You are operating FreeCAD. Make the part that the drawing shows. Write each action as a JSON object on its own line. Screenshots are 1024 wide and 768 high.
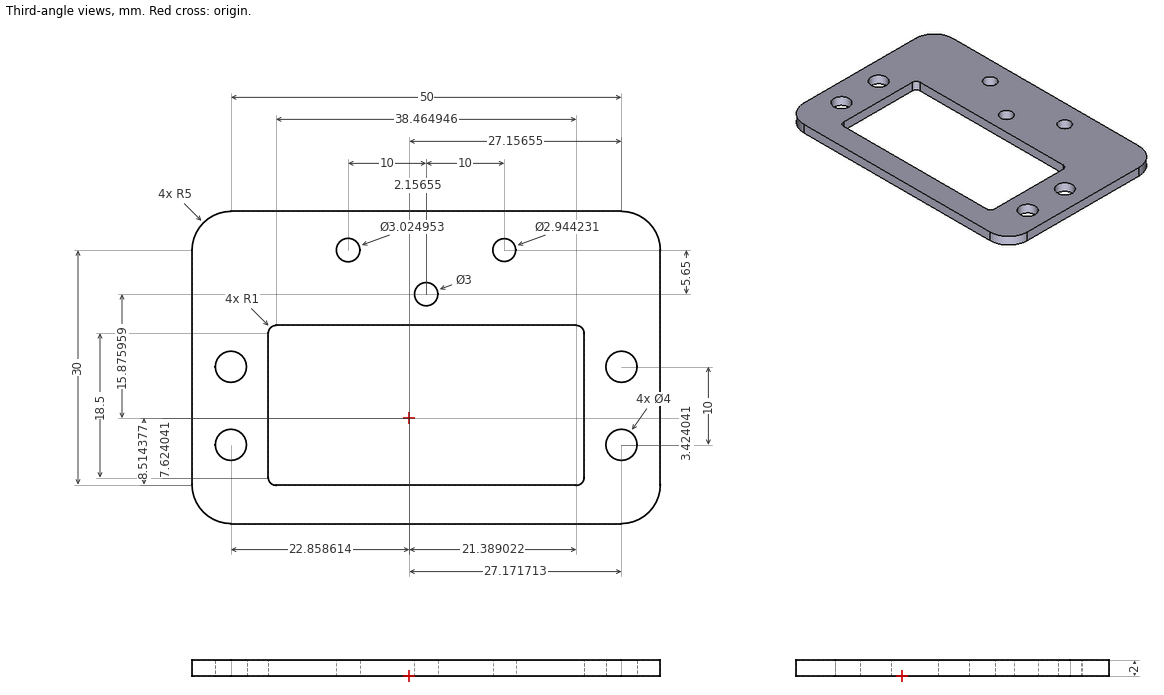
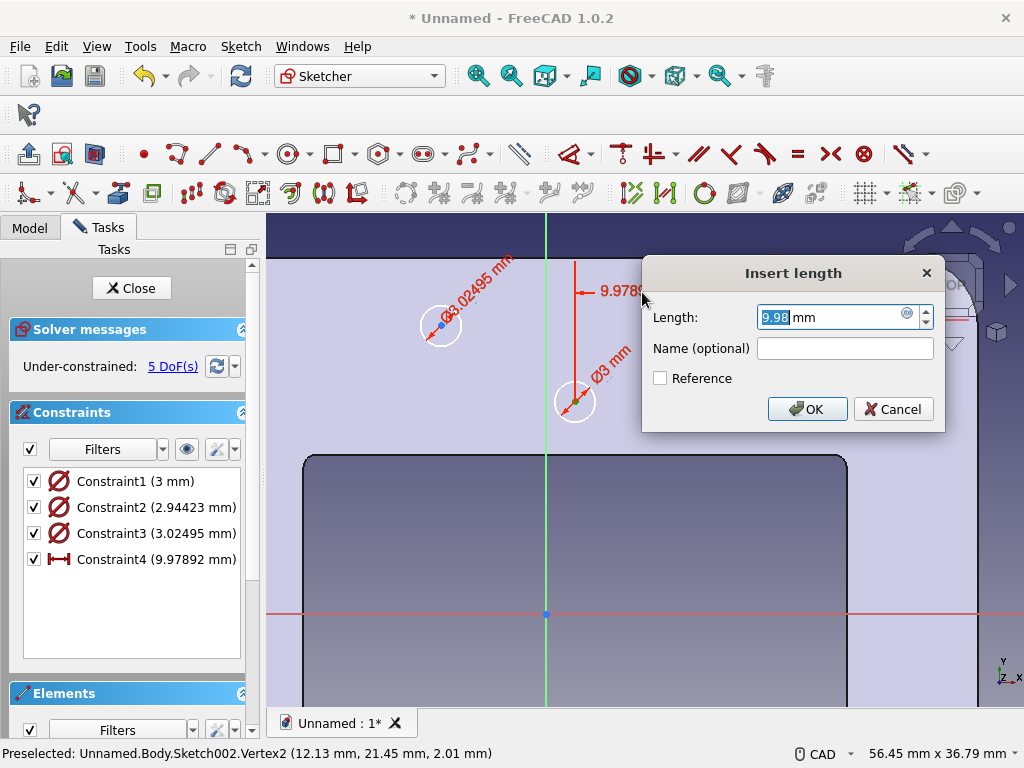
{"action": "type", "text": "10"}
{"action": "key", "text": "Return"}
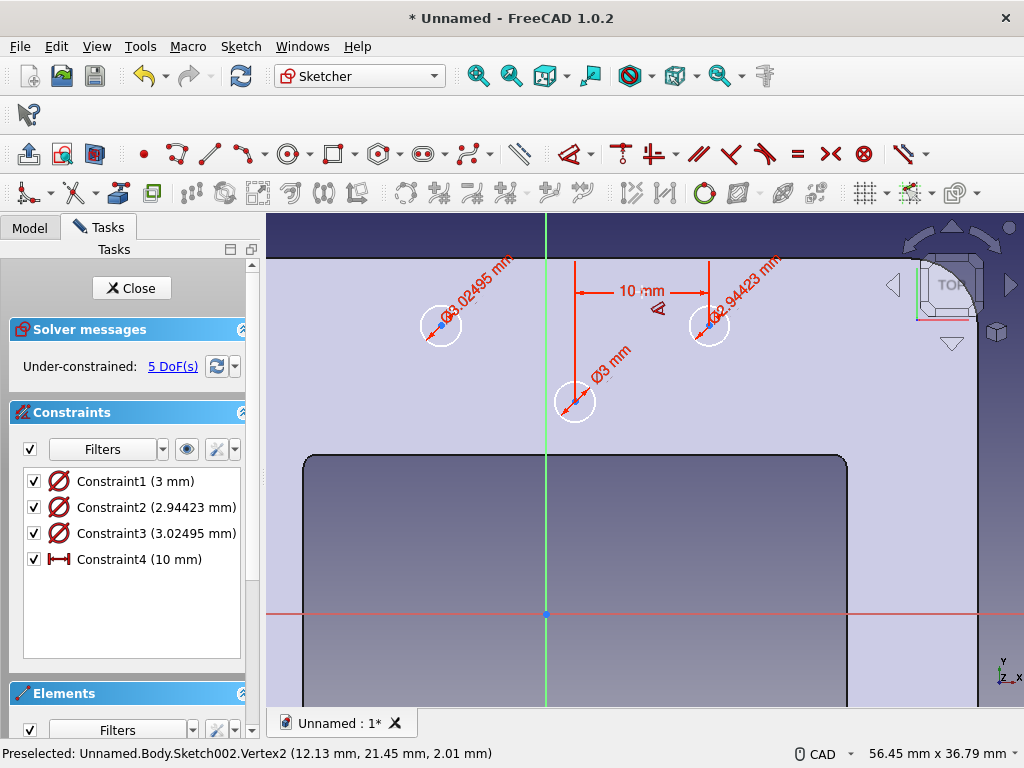
{"action": "left_click", "coordinate": [575, 402]}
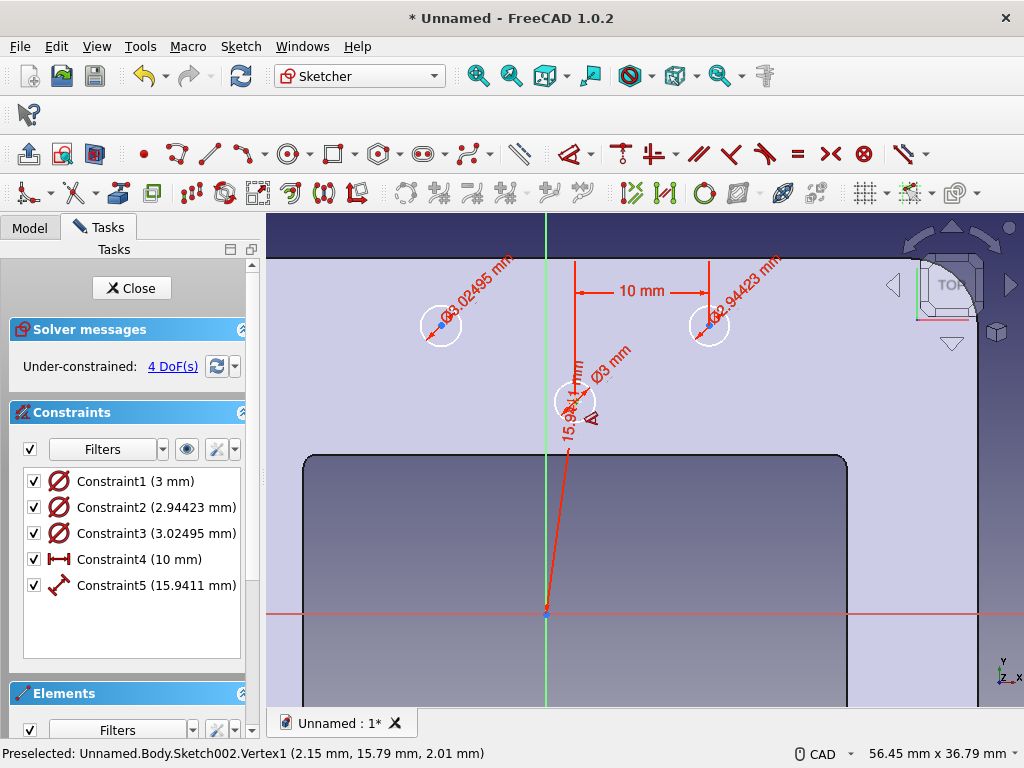
{"action": "left_click", "coordinate": [441, 326]}
{"action": "left_click", "coordinate": [508, 436]}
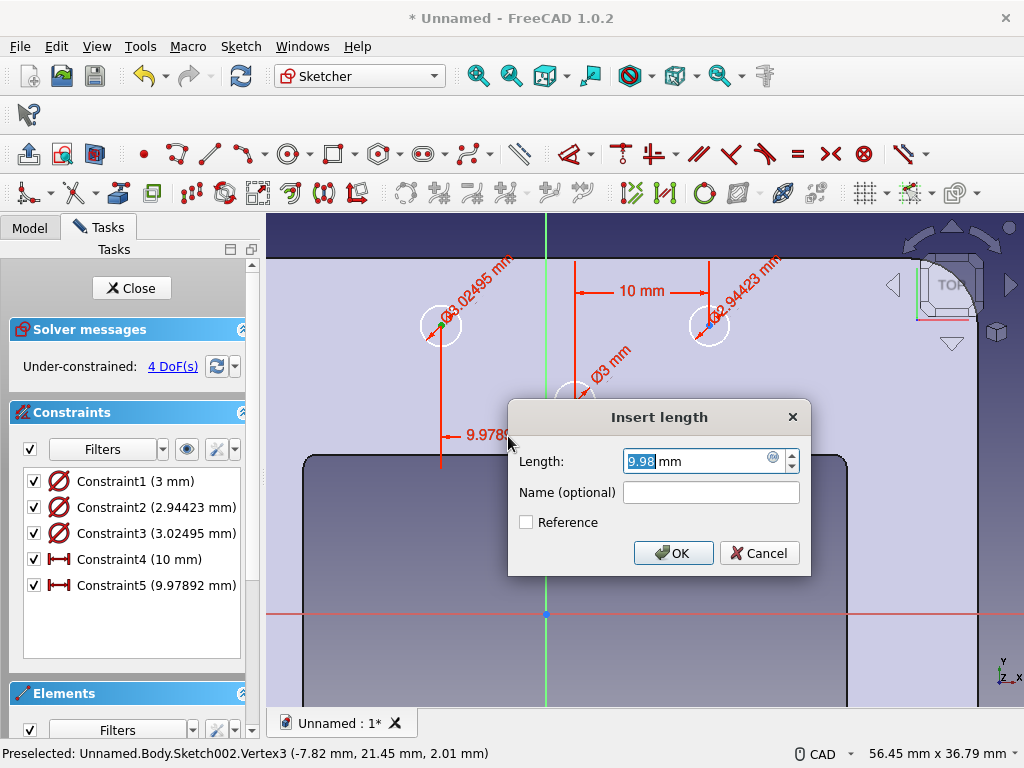
{"action": "type", "text": "10"}
{"action": "key", "text": "Return"}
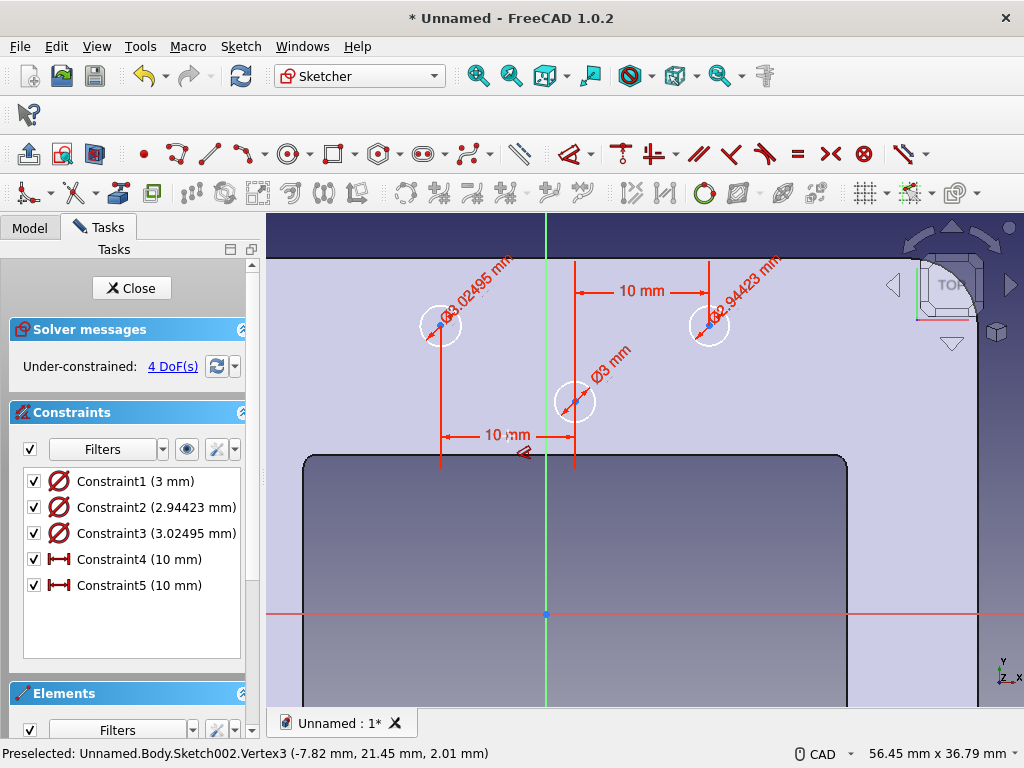
{"action": "left_click", "coordinate": [575, 402]}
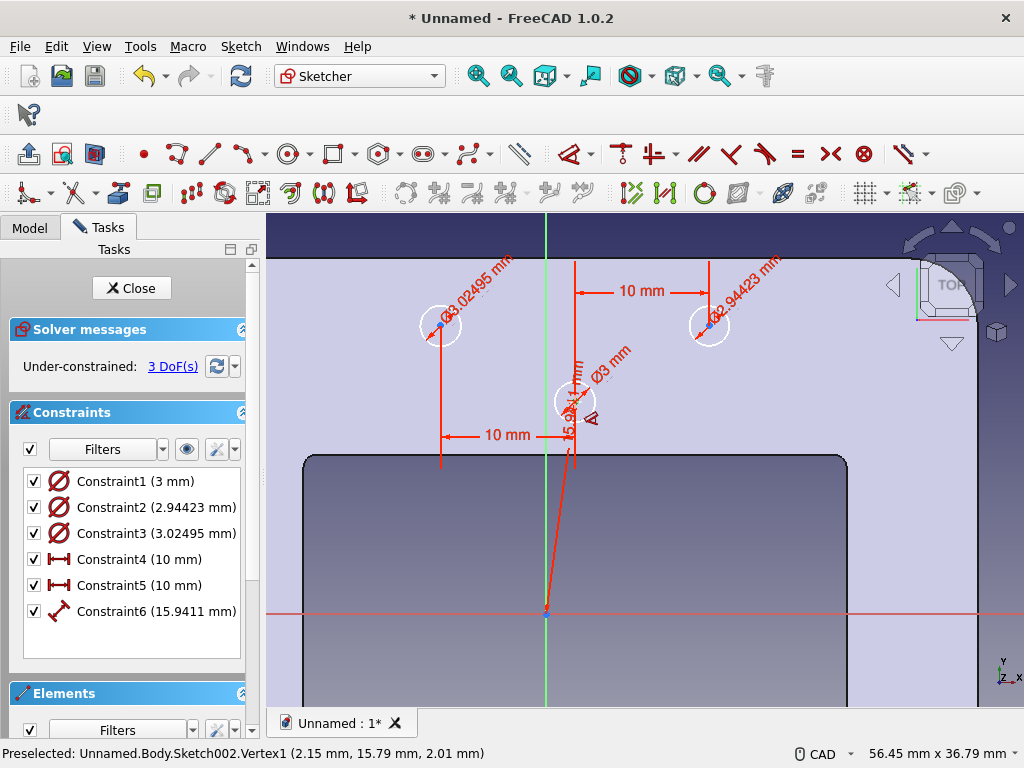
{"action": "left_click", "coordinate": [709, 326]}
{"action": "left_click", "coordinate": [743, 364]}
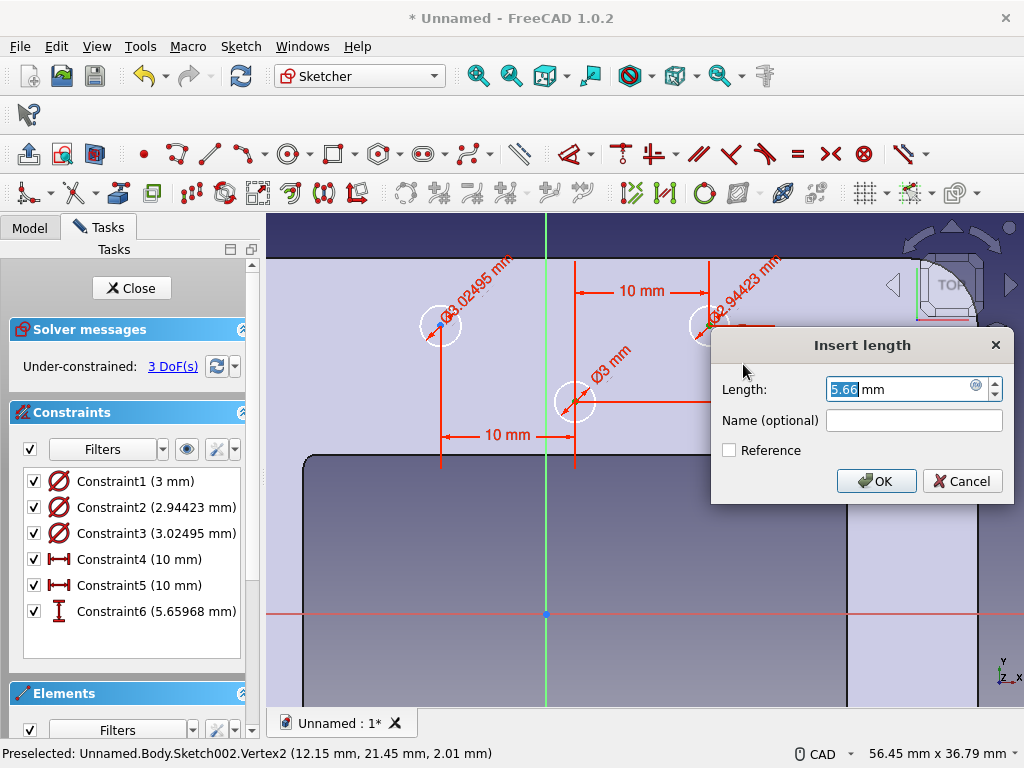
{"action": "type", "text": "5.65"}
{"action": "key", "text": "Return"}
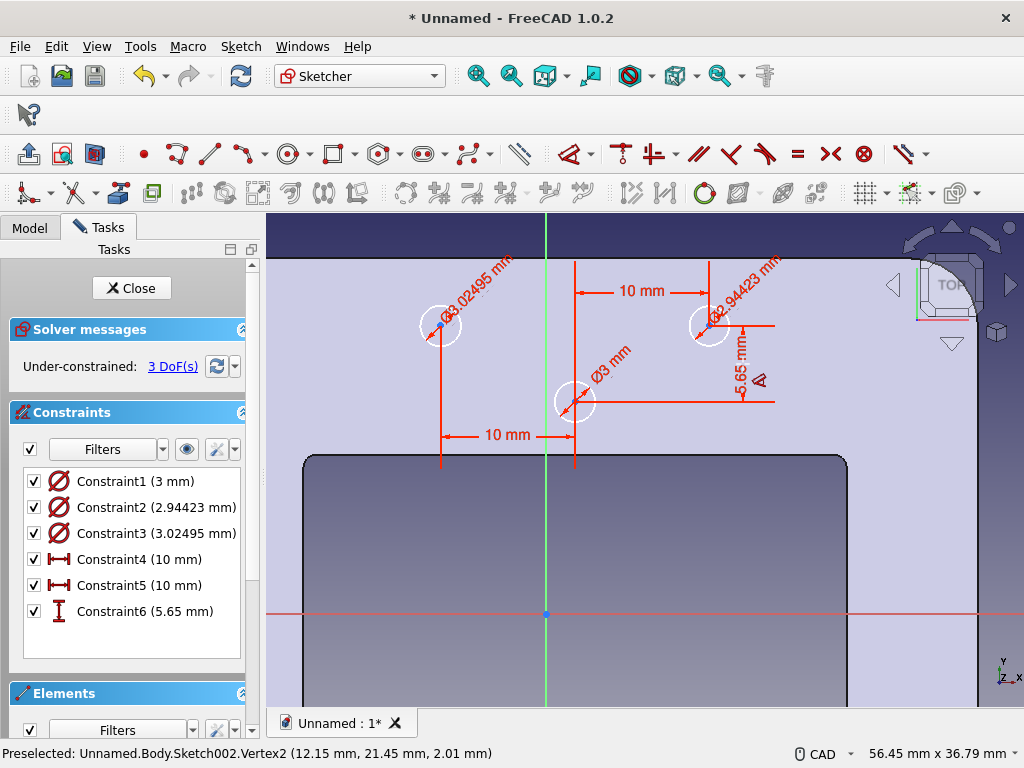
{"action": "left_click", "coordinate": [575, 402]}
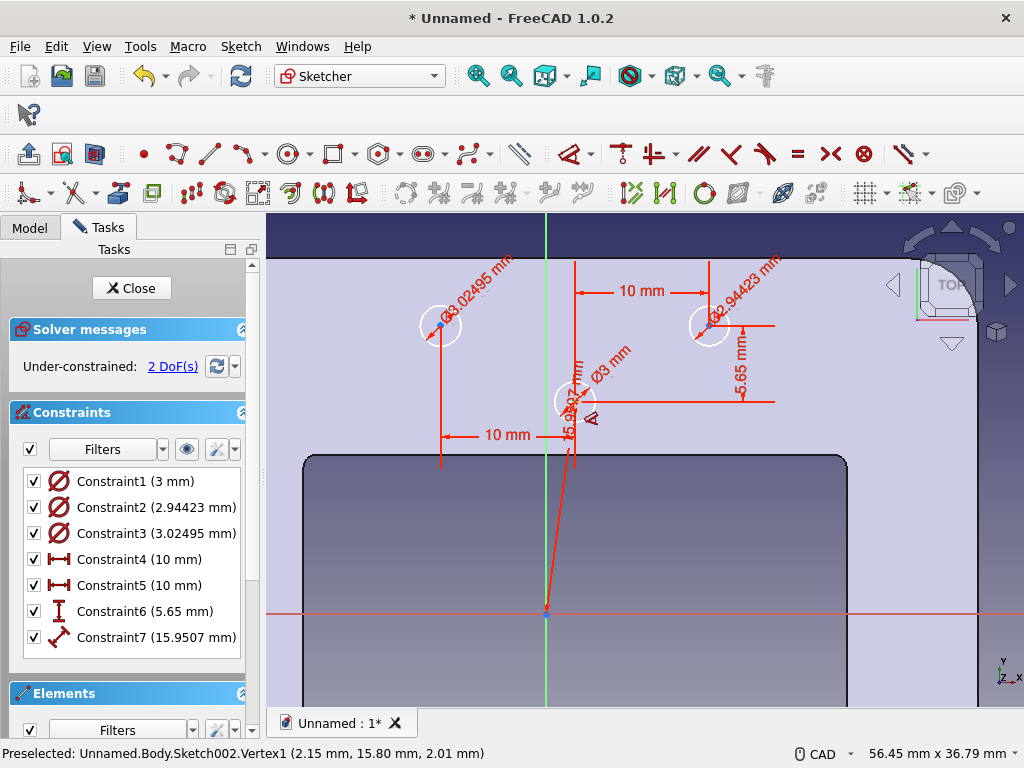
{"action": "left_click", "coordinate": [441, 326]}
{"action": "left_click", "coordinate": [407, 364]}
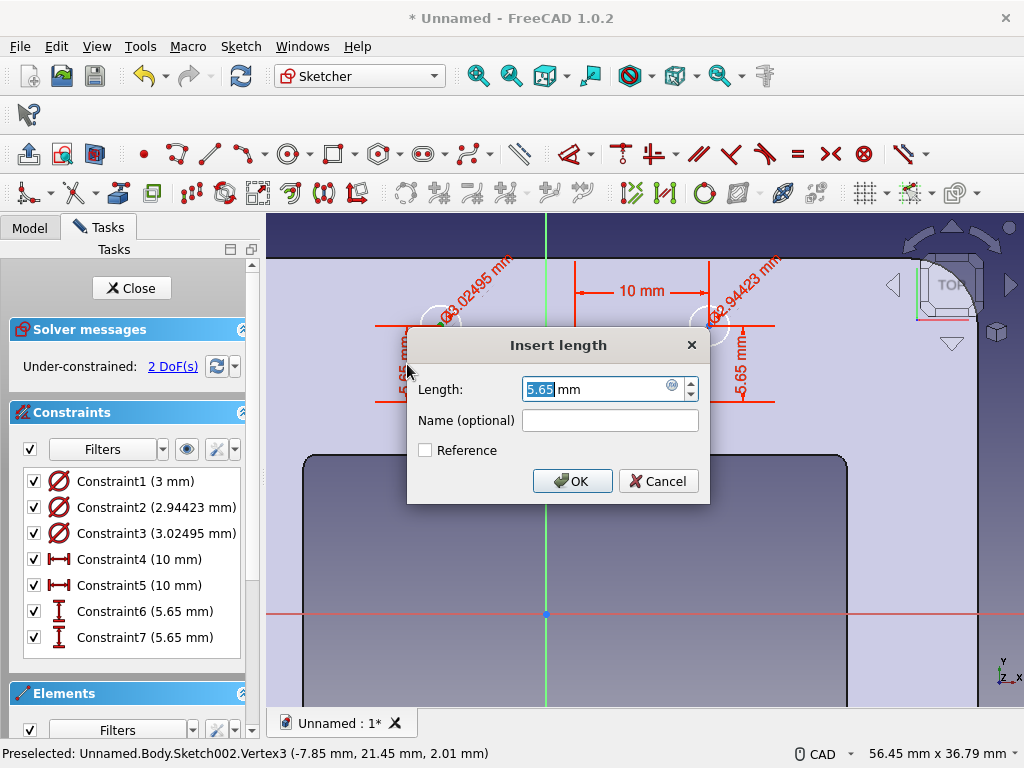
{"action": "type", "text": "5.65"}
{"action": "key", "text": "Return"}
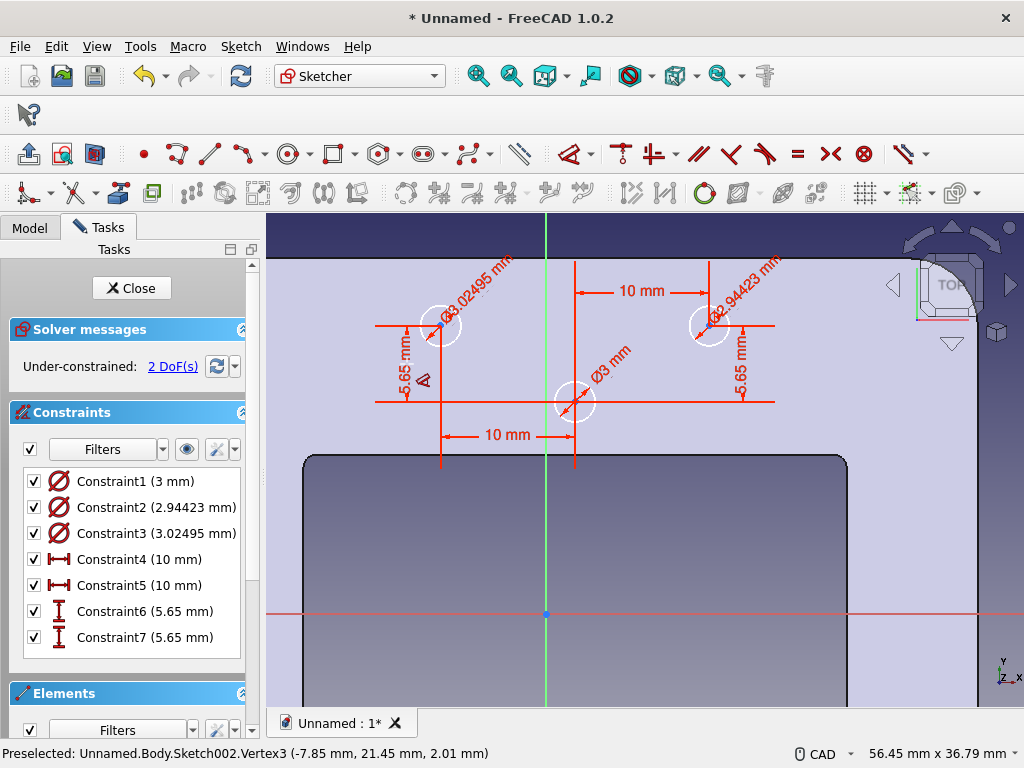
{"action": "scroll", "coordinate": [575, 402], "scroll_direction": "up", "scroll_amount": 2}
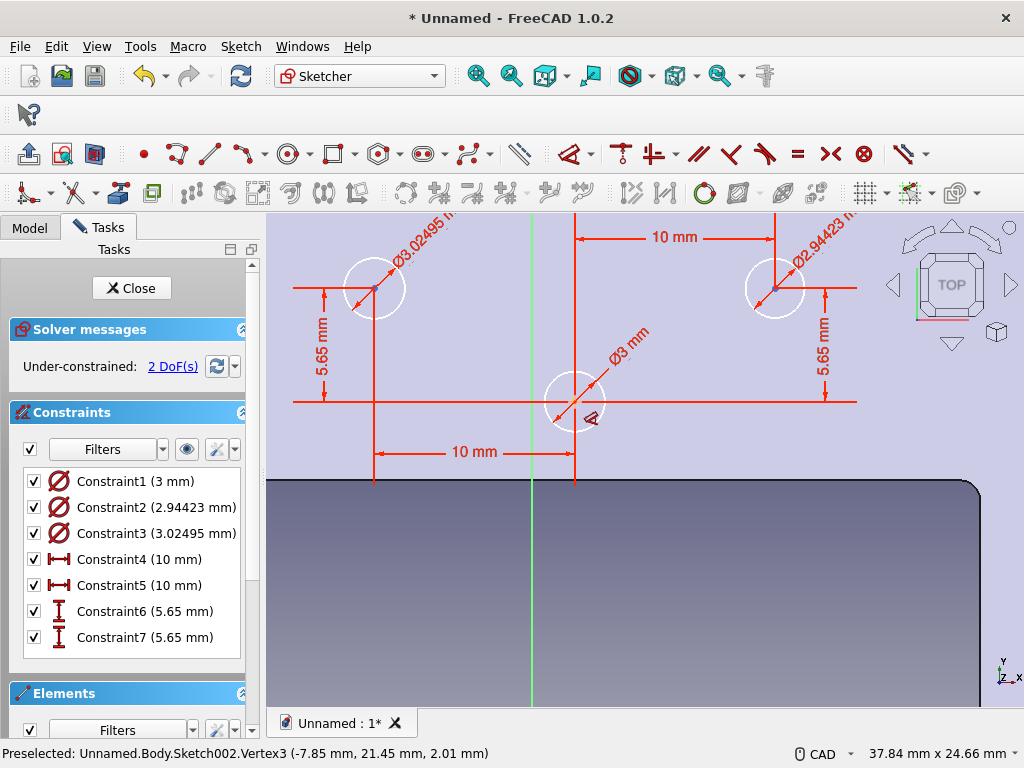
{"action": "left_click", "coordinate": [575, 402]}
{"action": "left_click", "coordinate": [553, 344]}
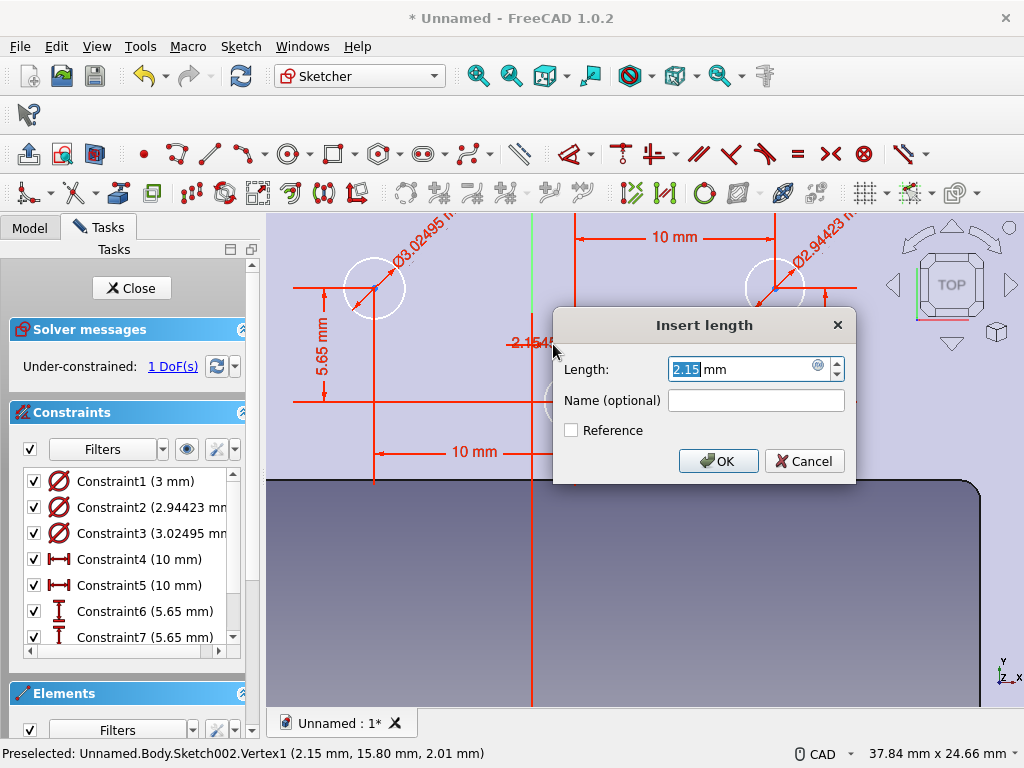
{"action": "type", "text": "2.15655"}
{"action": "key", "text": "Return"}